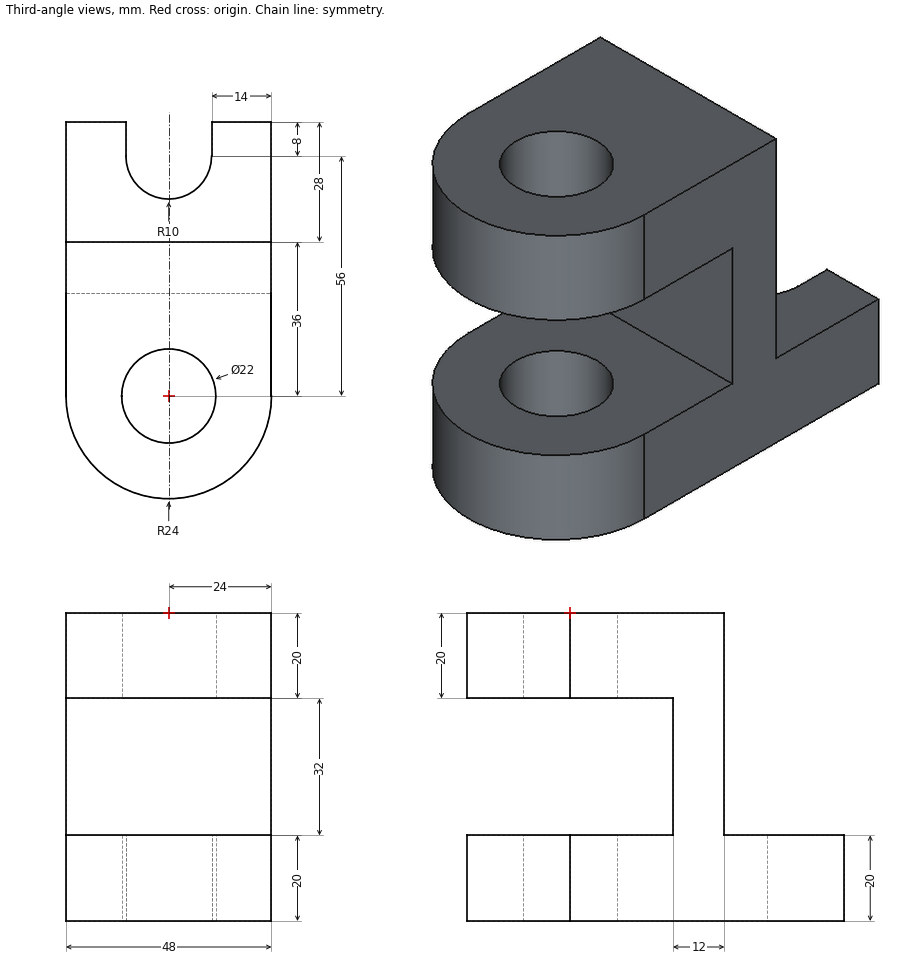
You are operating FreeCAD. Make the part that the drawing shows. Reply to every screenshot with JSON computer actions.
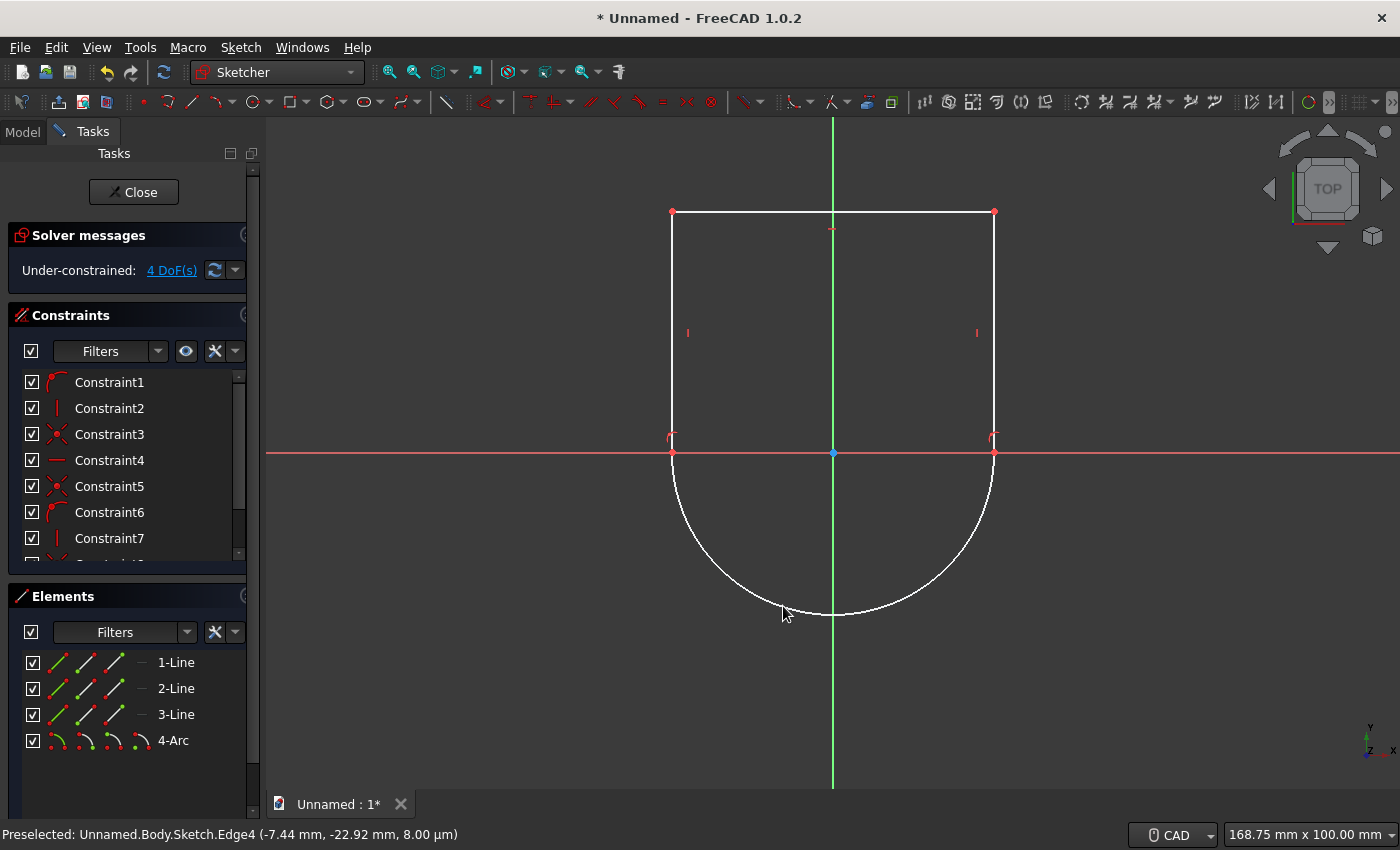
{"action": "left_click", "coordinate": [994, 381]}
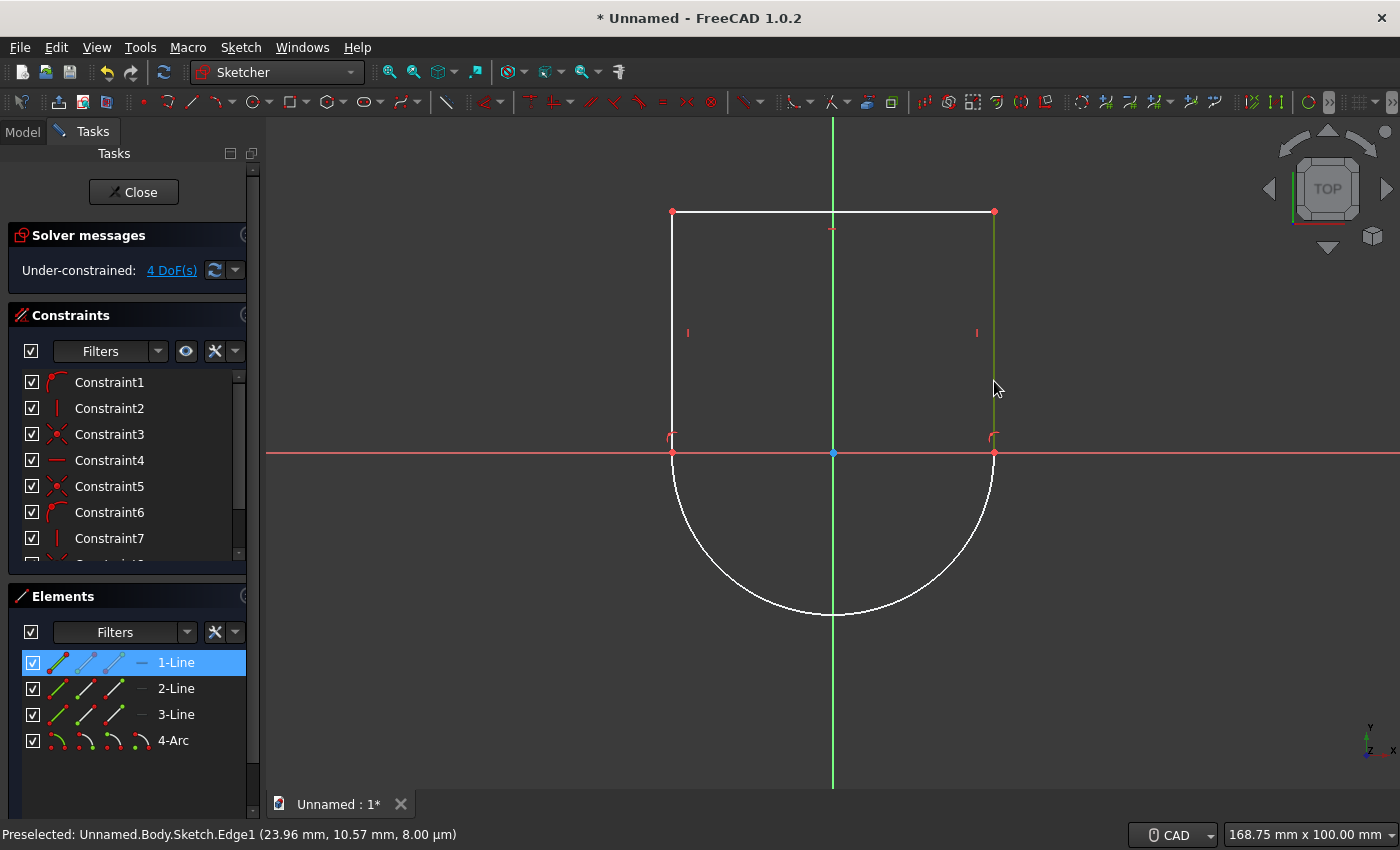
{"action": "left_click", "coordinate": [738, 584]}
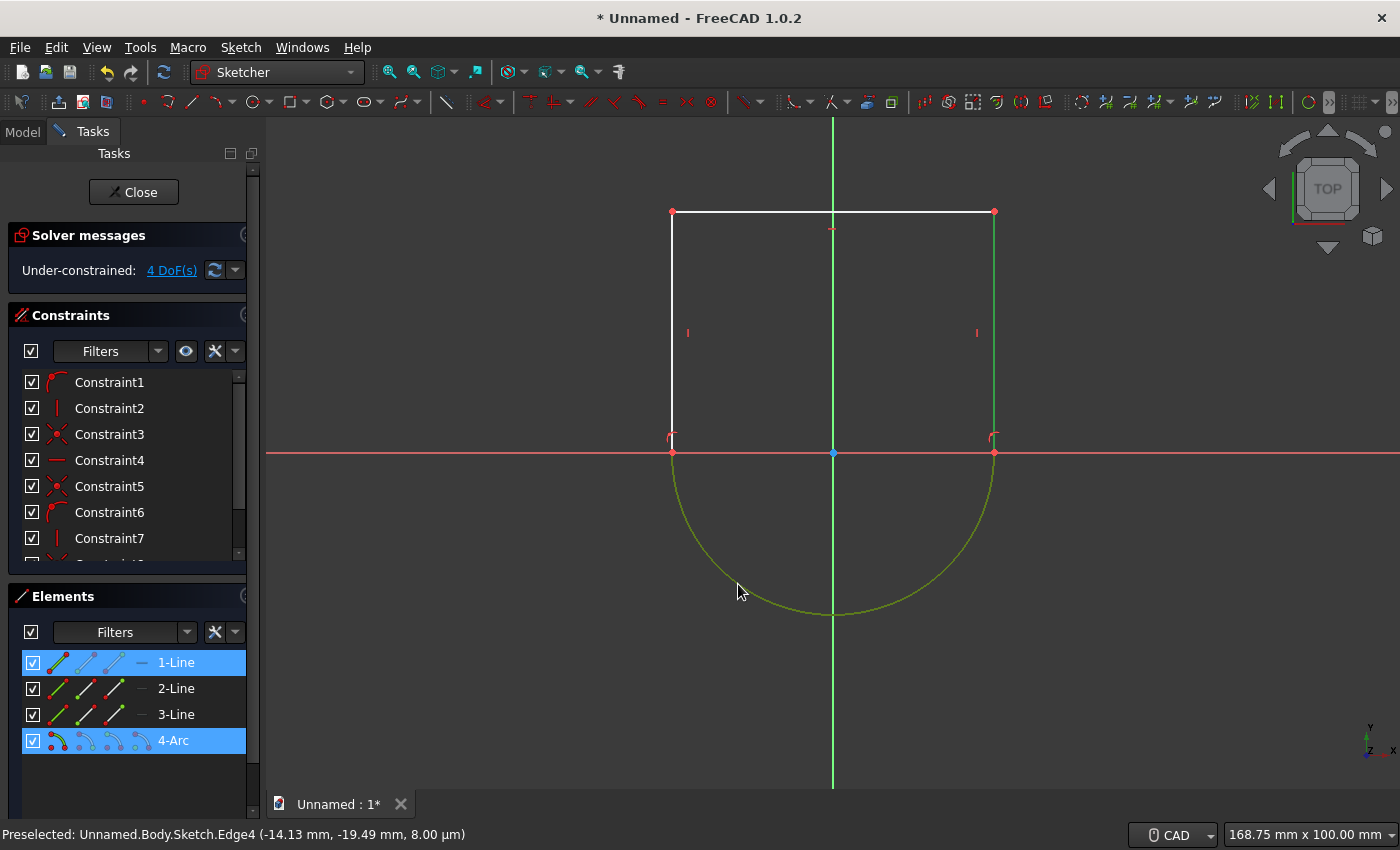
{"action": "left_click", "coordinate": [640, 102]}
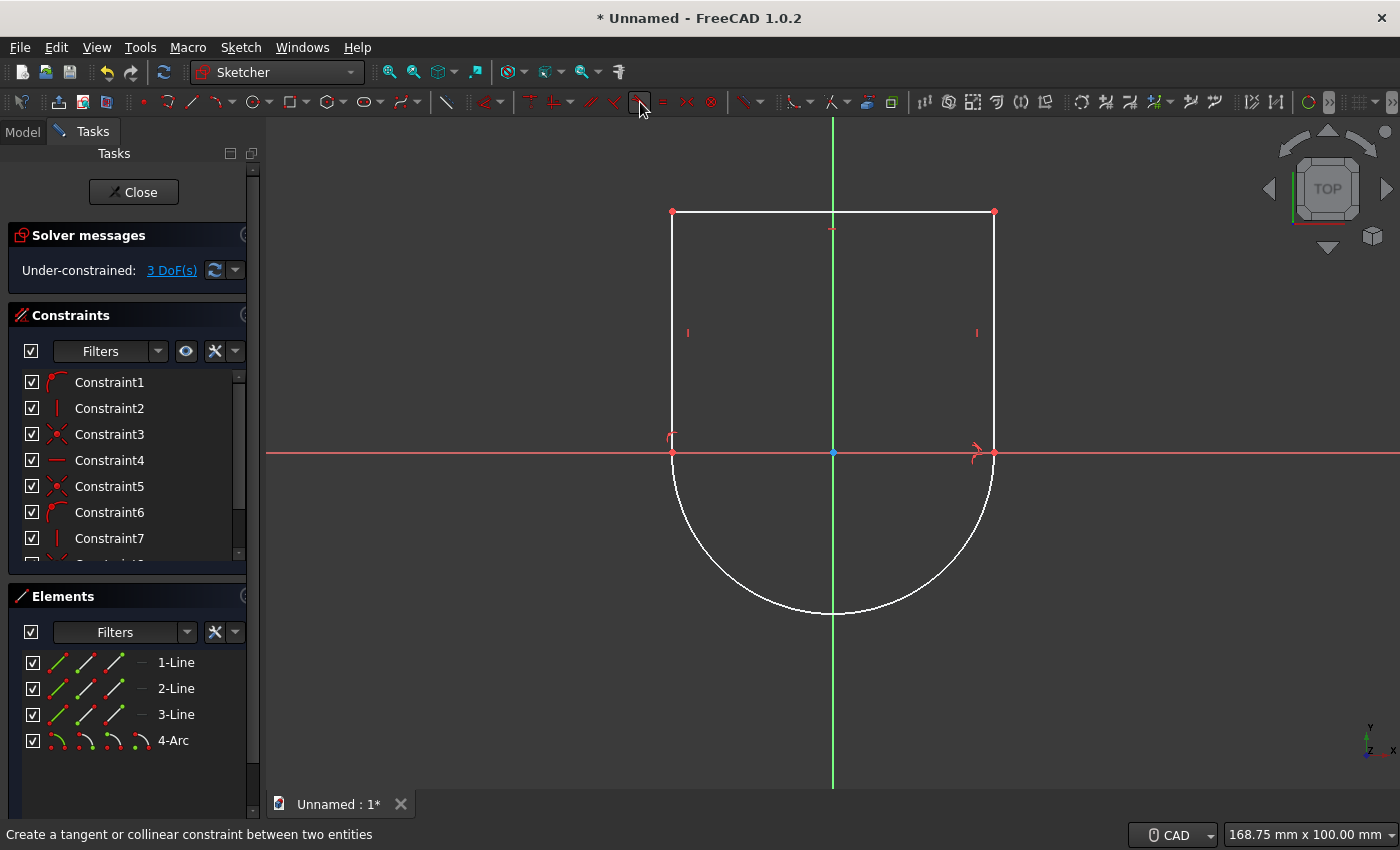
{"action": "left_click", "coordinate": [833, 453]}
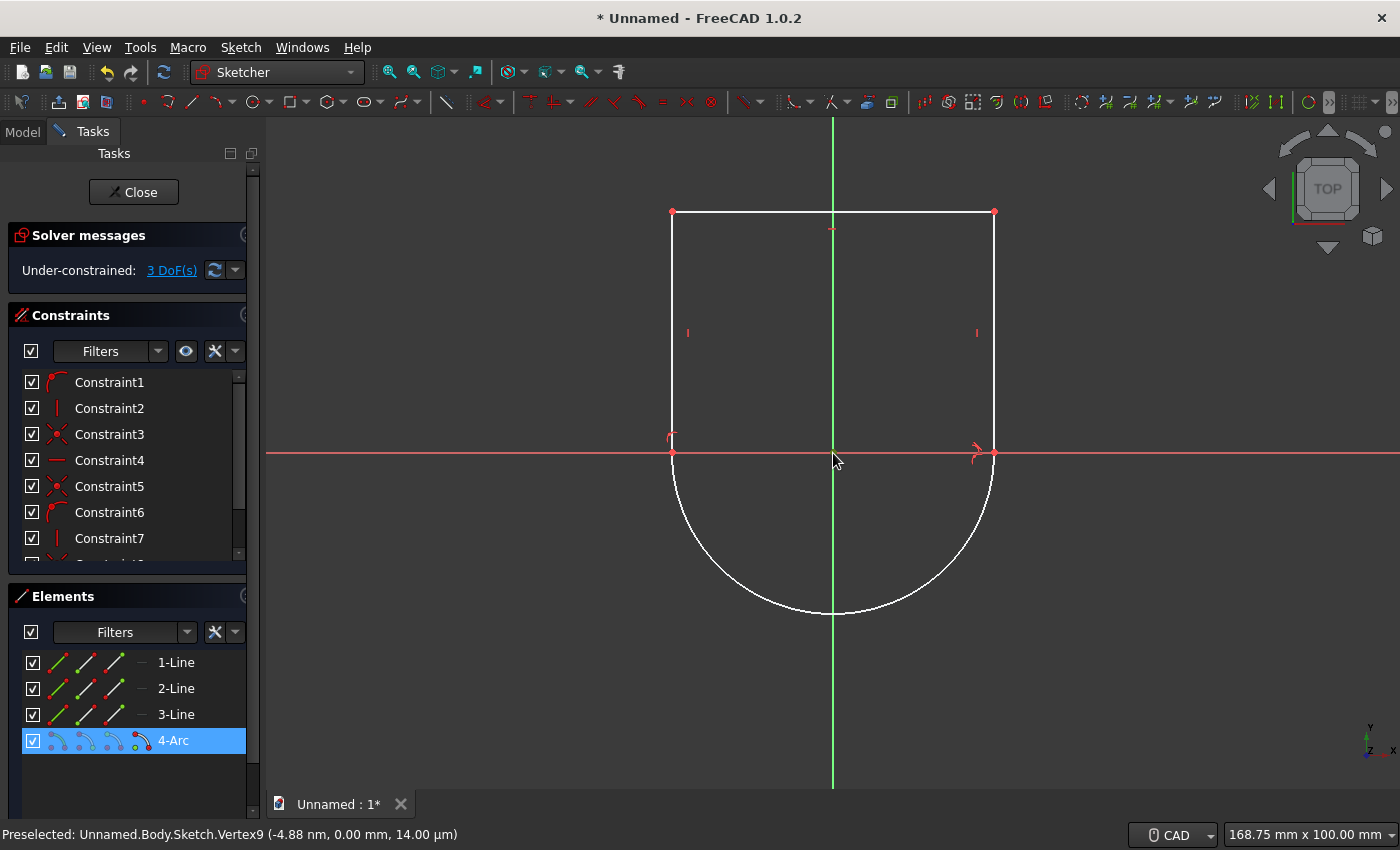
{"action": "left_click", "coordinate": [833, 717]}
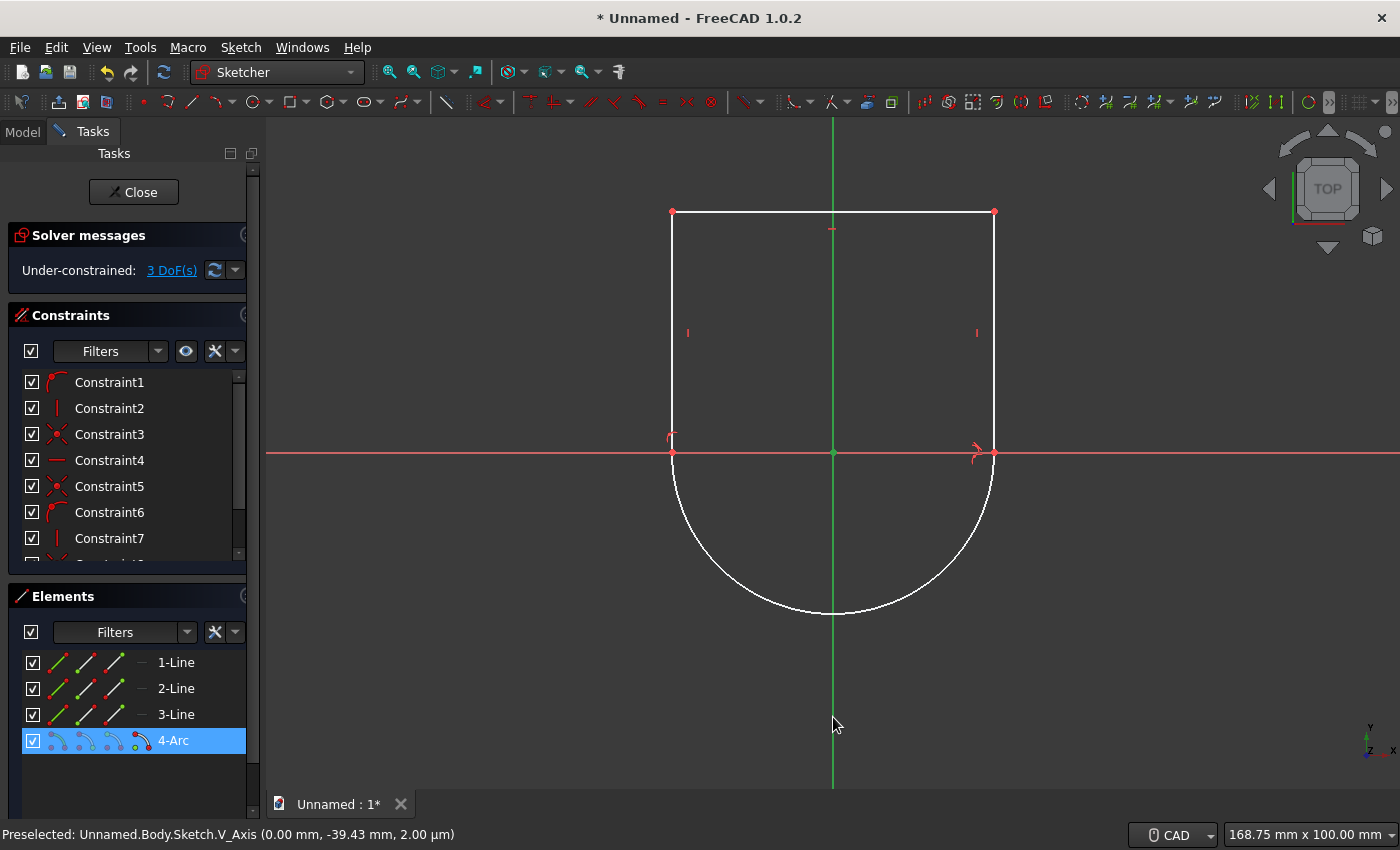
{"action": "left_click", "coordinate": [530, 102]}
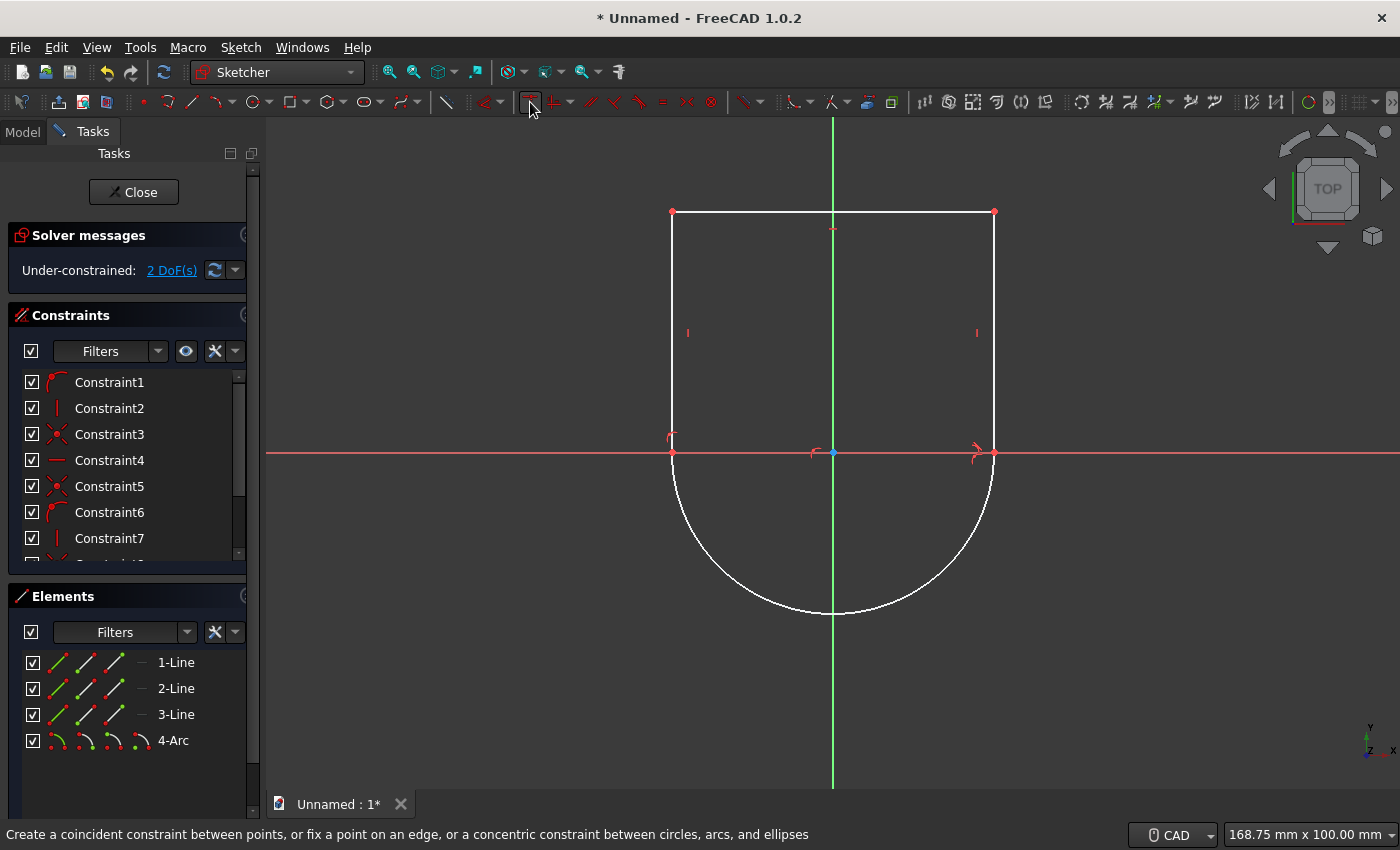
{"action": "left_click", "coordinate": [738, 583]}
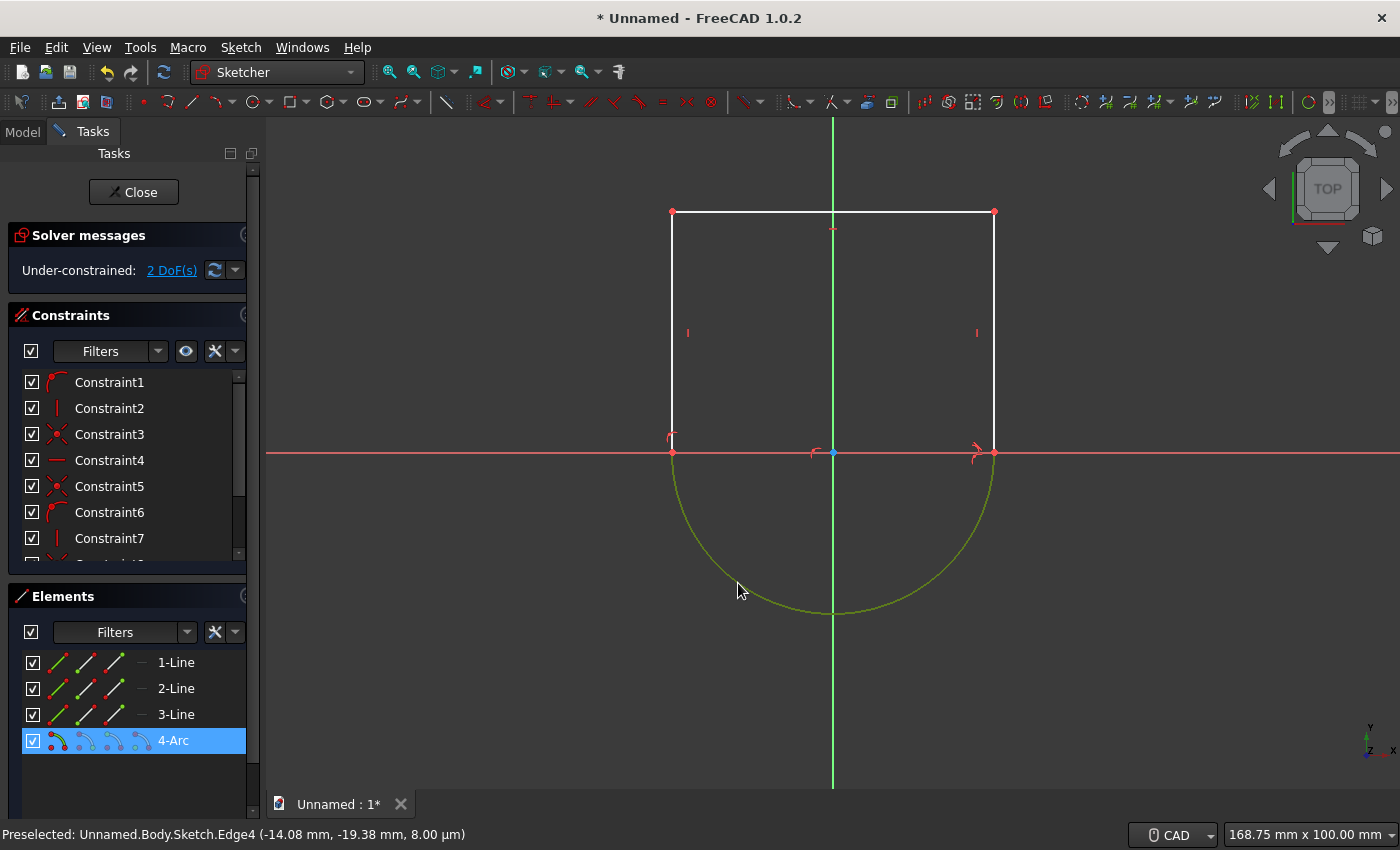
{"action": "key", "text": "k r"}